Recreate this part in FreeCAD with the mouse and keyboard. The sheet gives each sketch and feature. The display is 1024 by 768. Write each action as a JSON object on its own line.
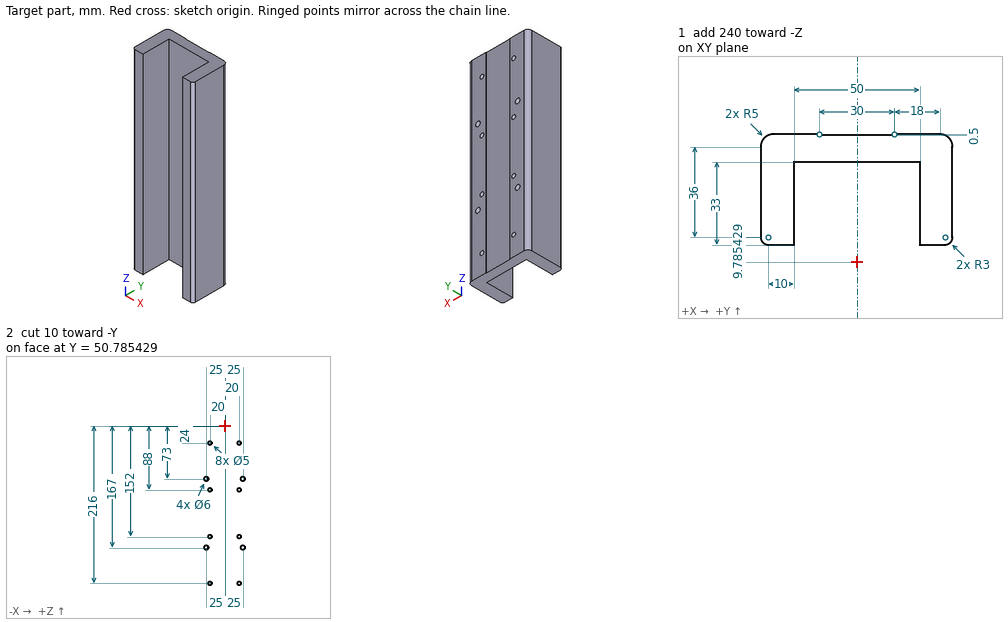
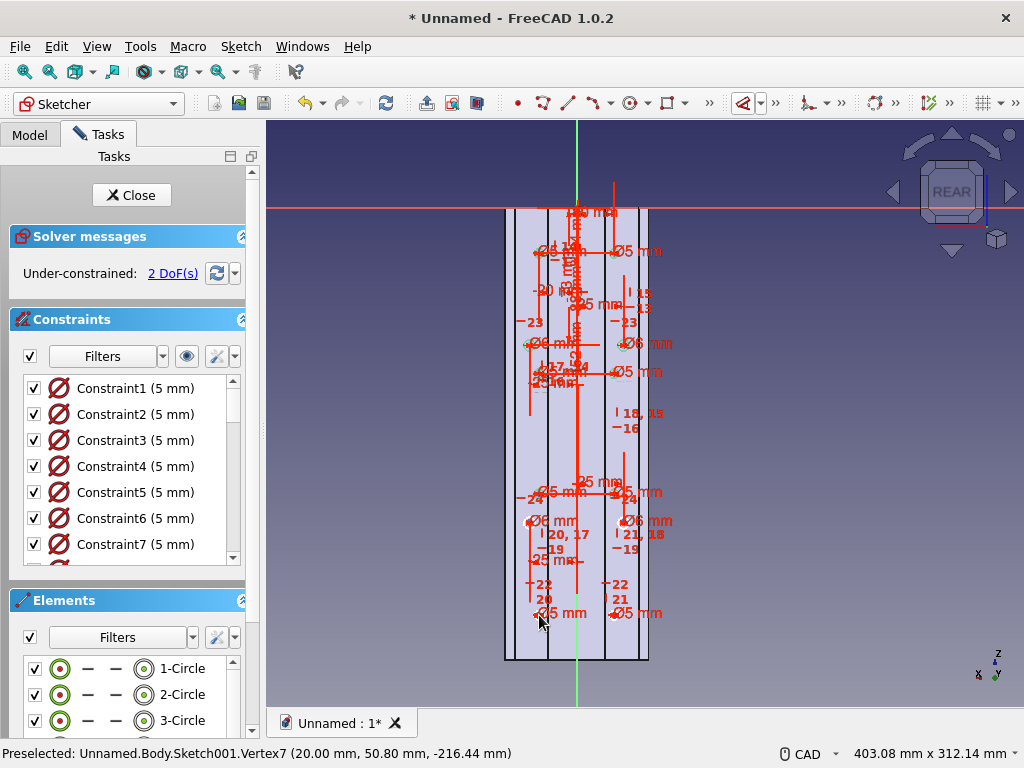
{"action": "key", "text": "i"}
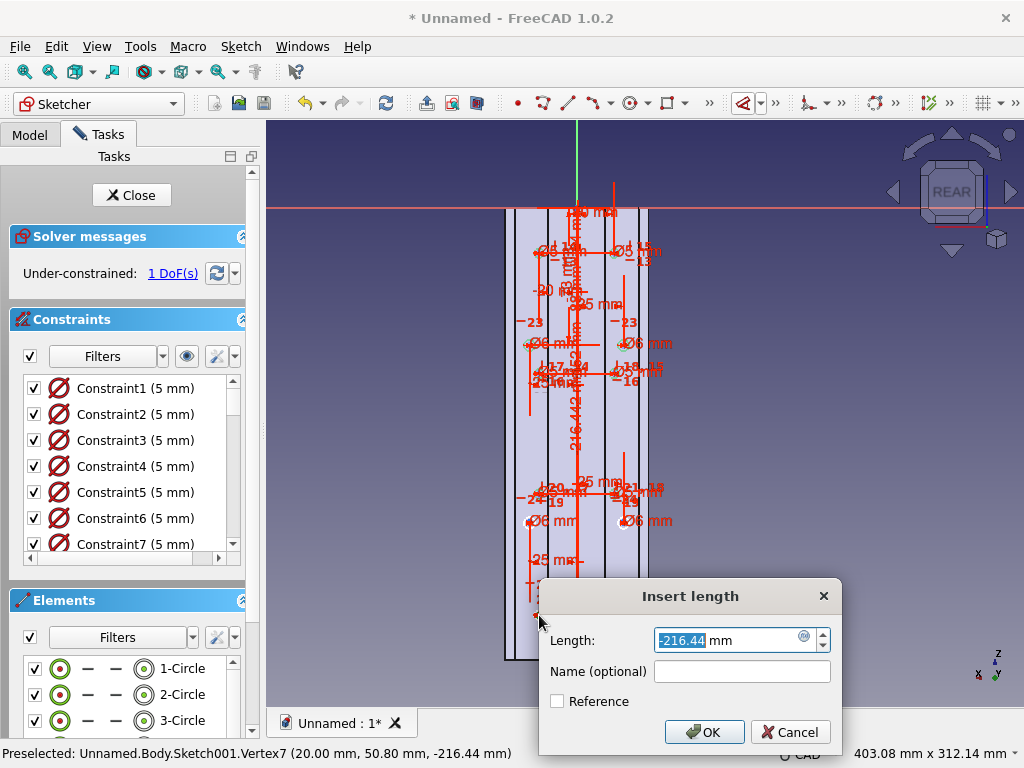
{"action": "type", "text": "-216"}
{"action": "key", "text": "Return"}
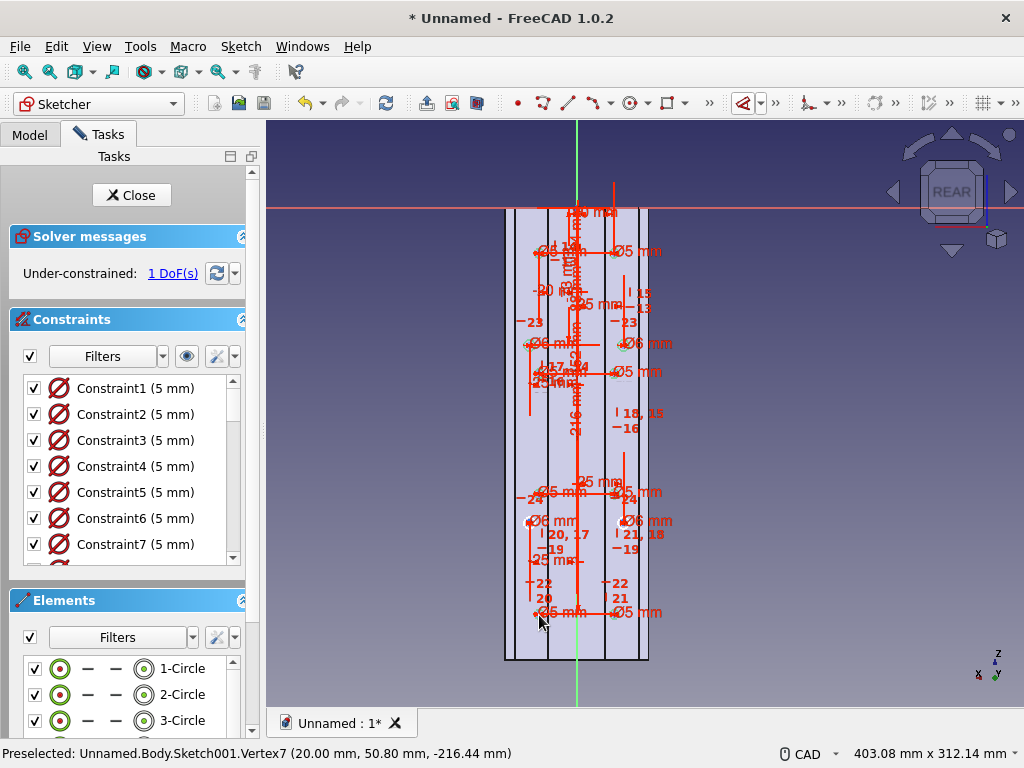
{"action": "left_click", "coordinate": [530, 523]}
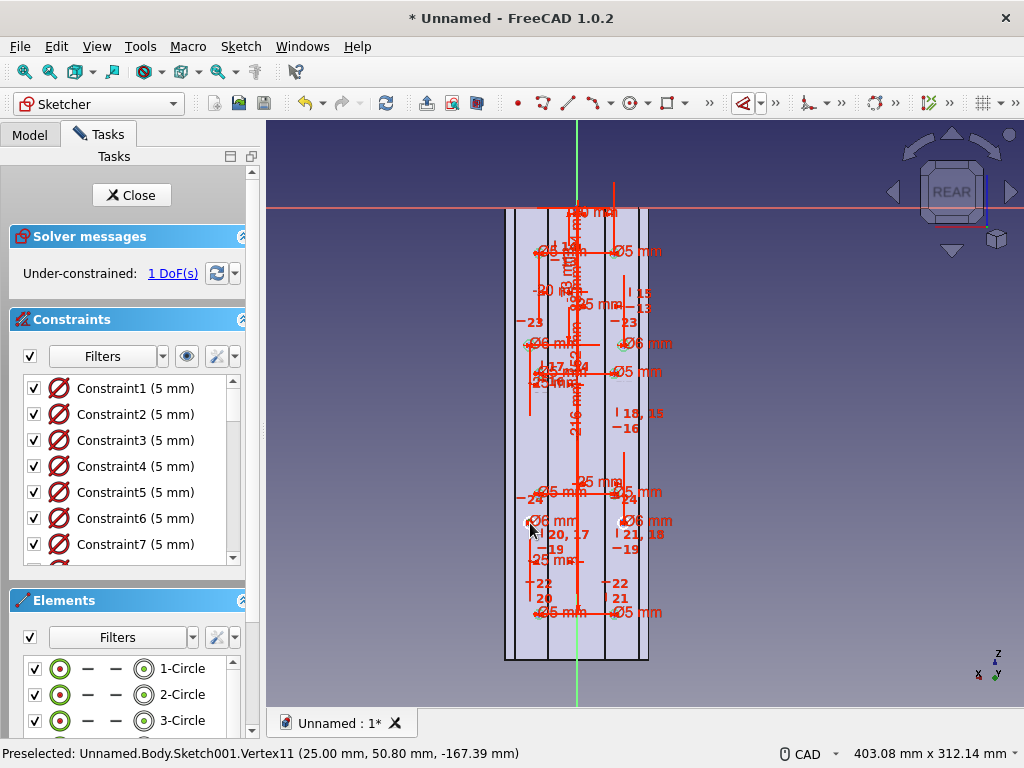
{"action": "key", "text": "i"}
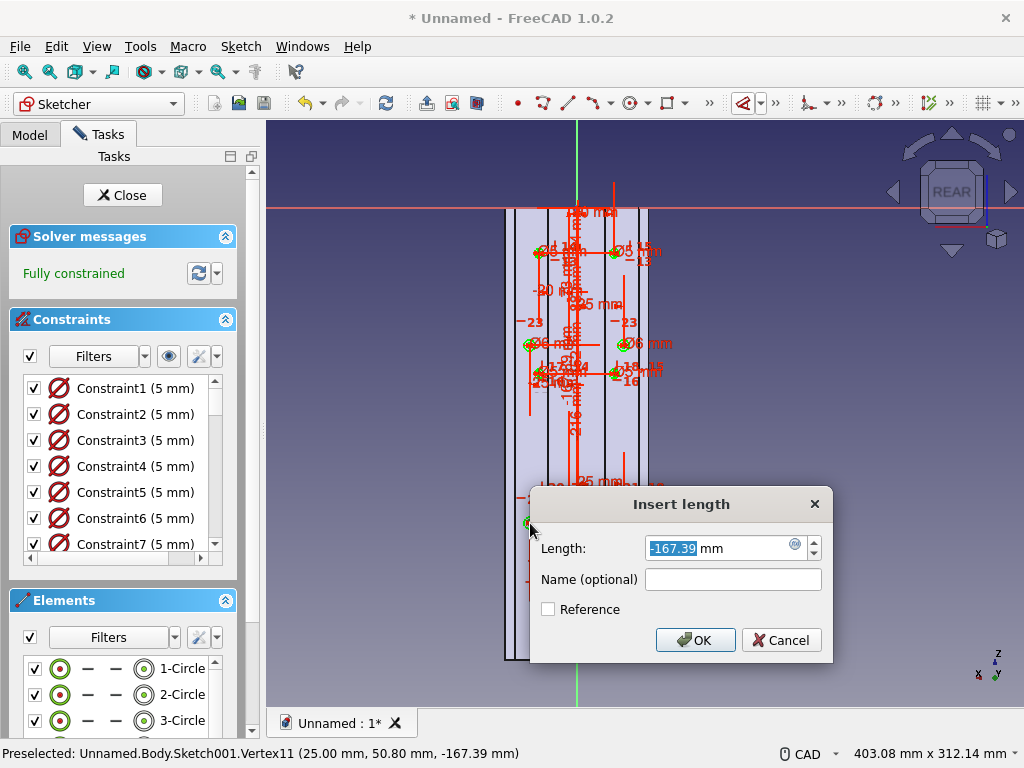
{"action": "type", "text": "-167"}
{"action": "key", "text": "Return"}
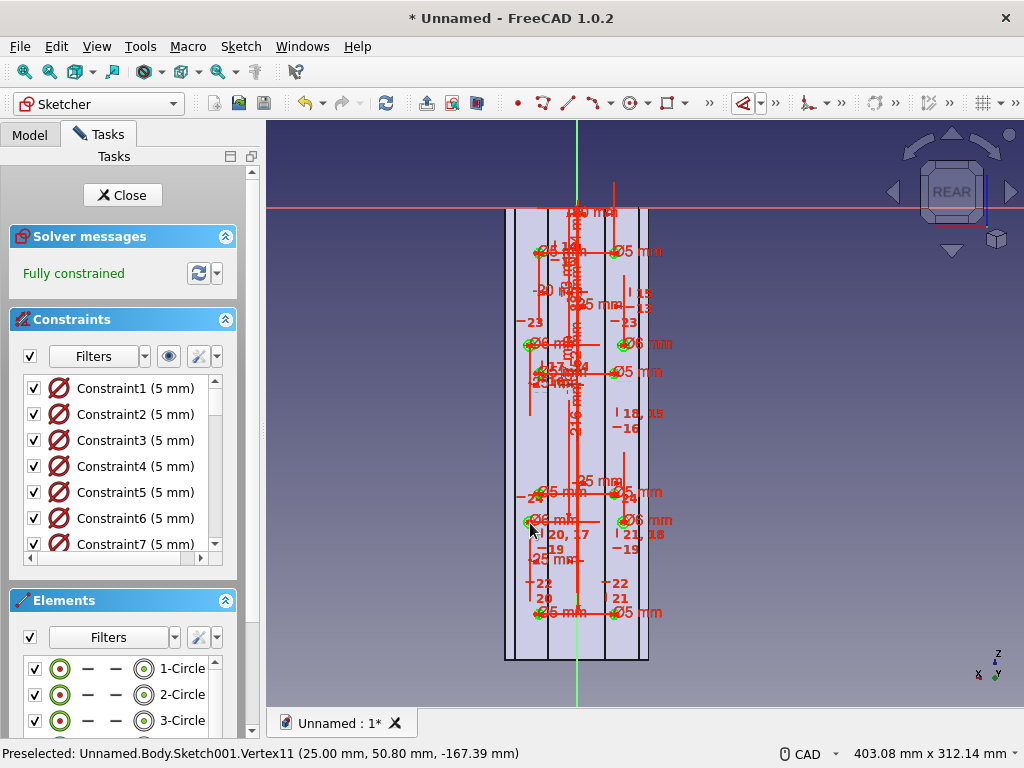
{"action": "left_click", "coordinate": [123, 195]}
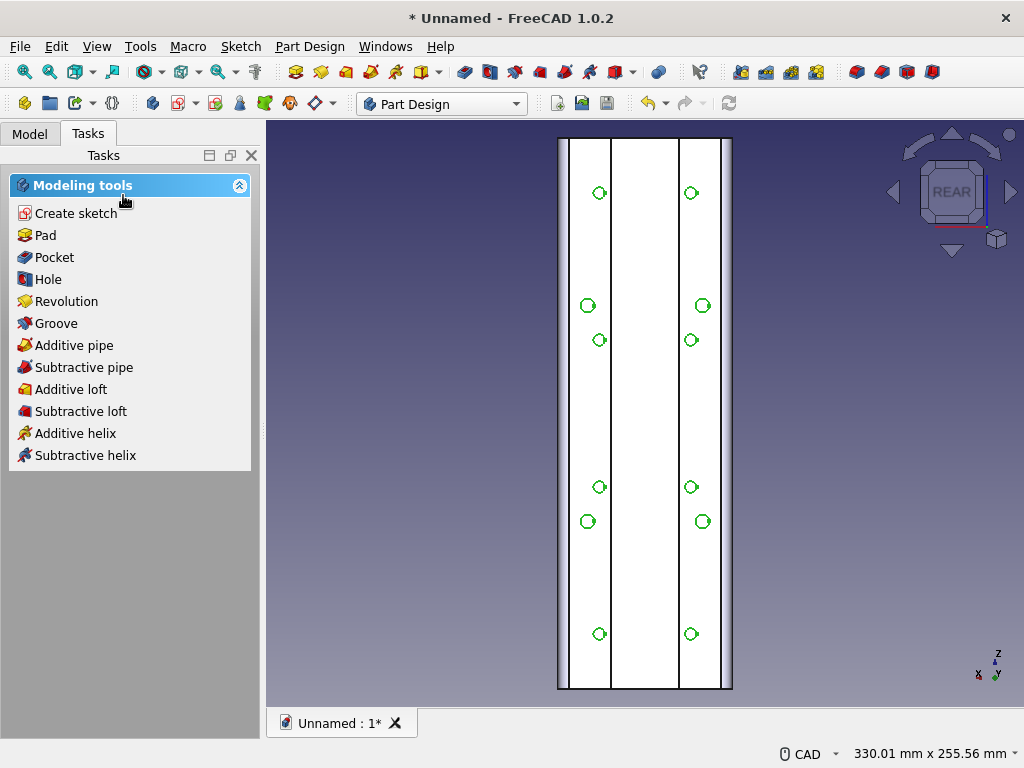
{"action": "left_click", "coordinate": [465, 72]}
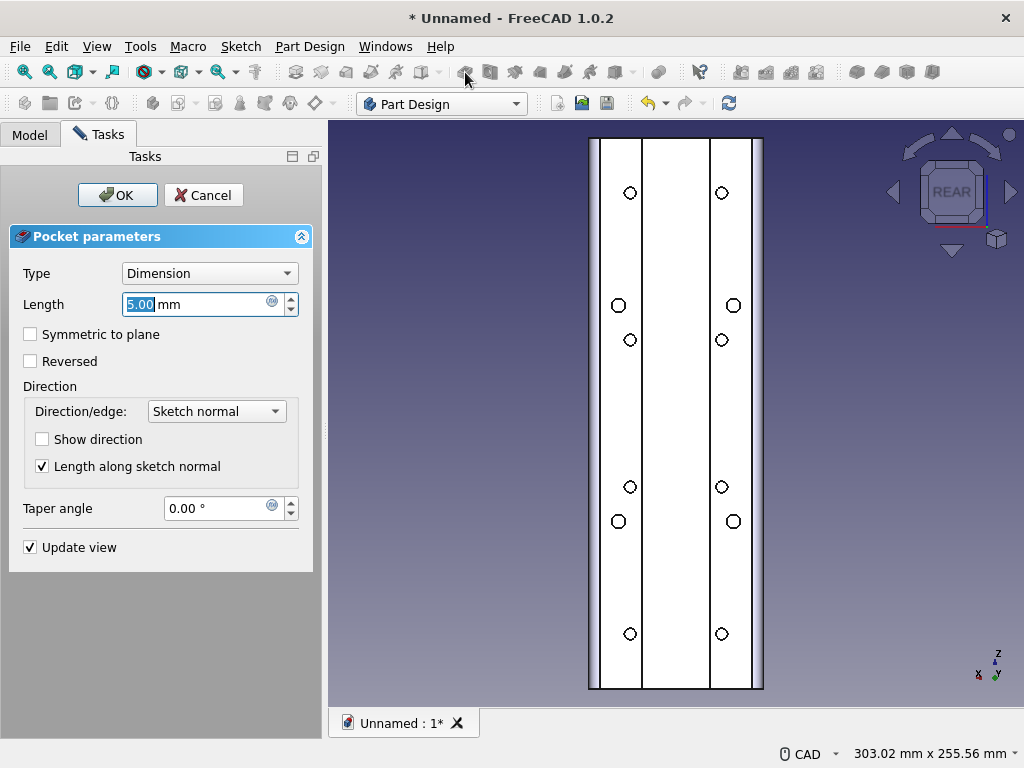
{"action": "type", "text": "10"}
{"action": "key", "text": "Tab"}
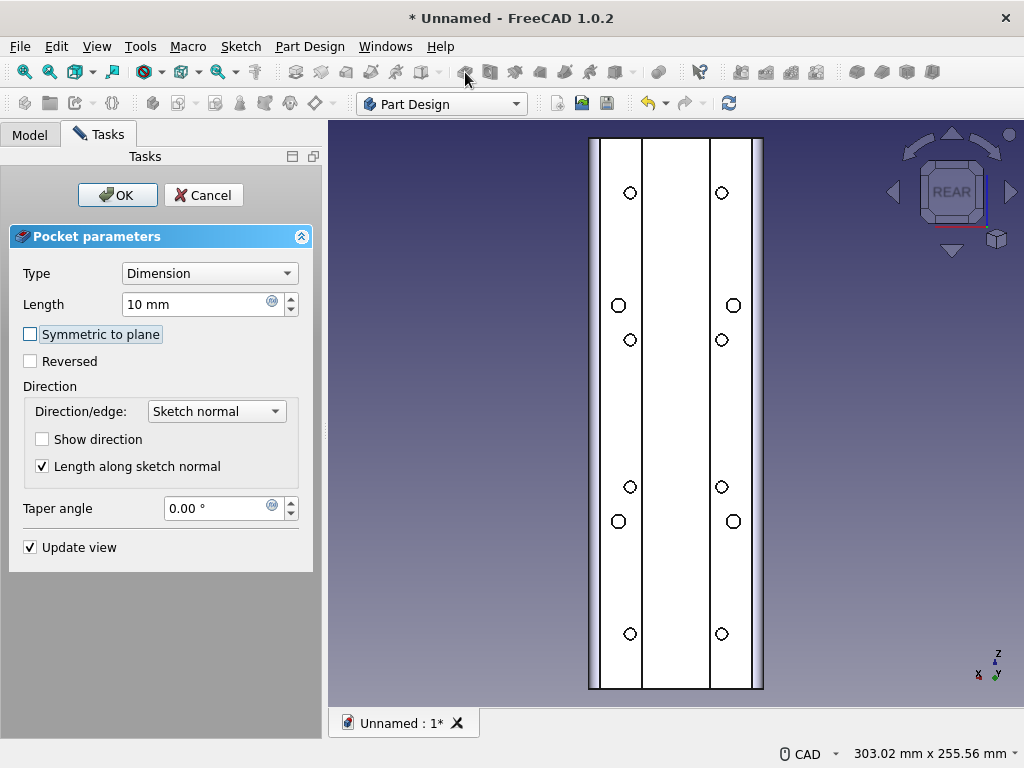
{"action": "left_click", "coordinate": [118, 195]}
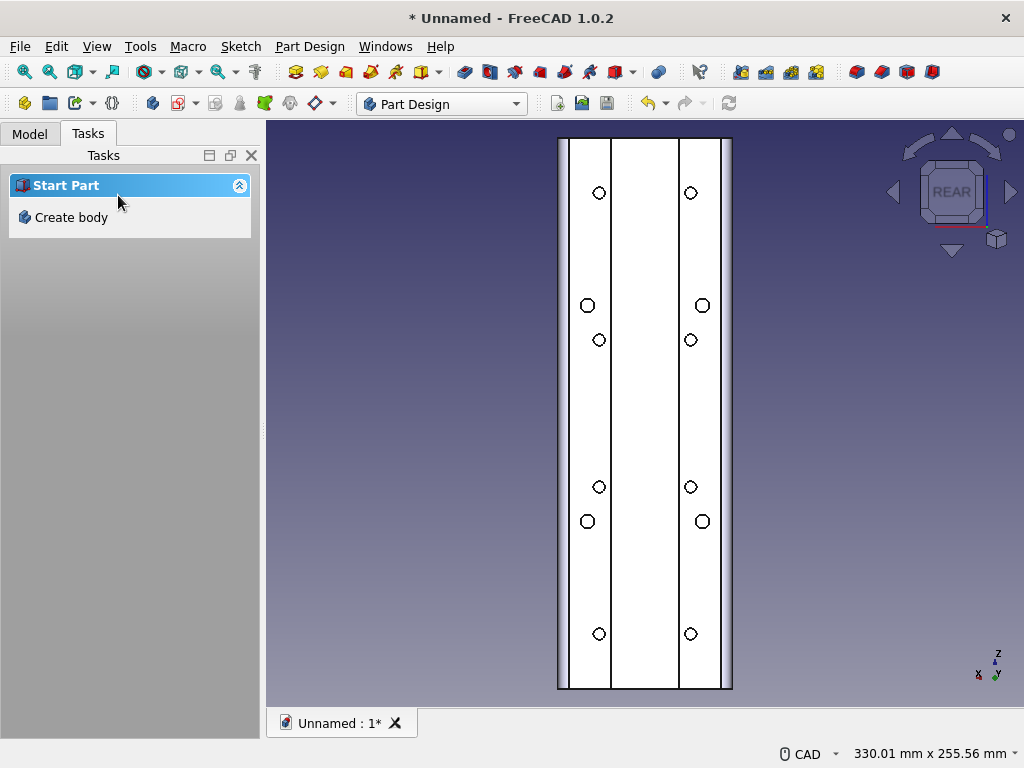
{"action": "key", "text": "0"}